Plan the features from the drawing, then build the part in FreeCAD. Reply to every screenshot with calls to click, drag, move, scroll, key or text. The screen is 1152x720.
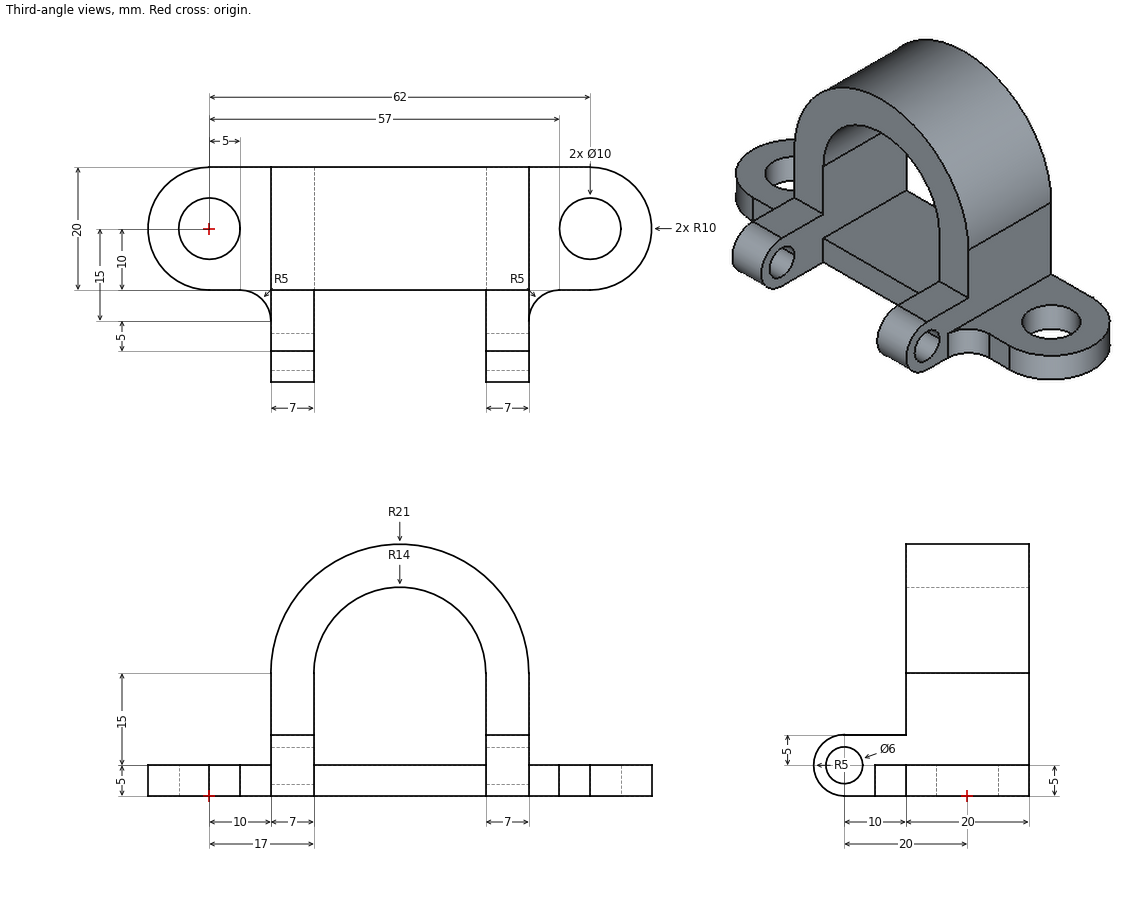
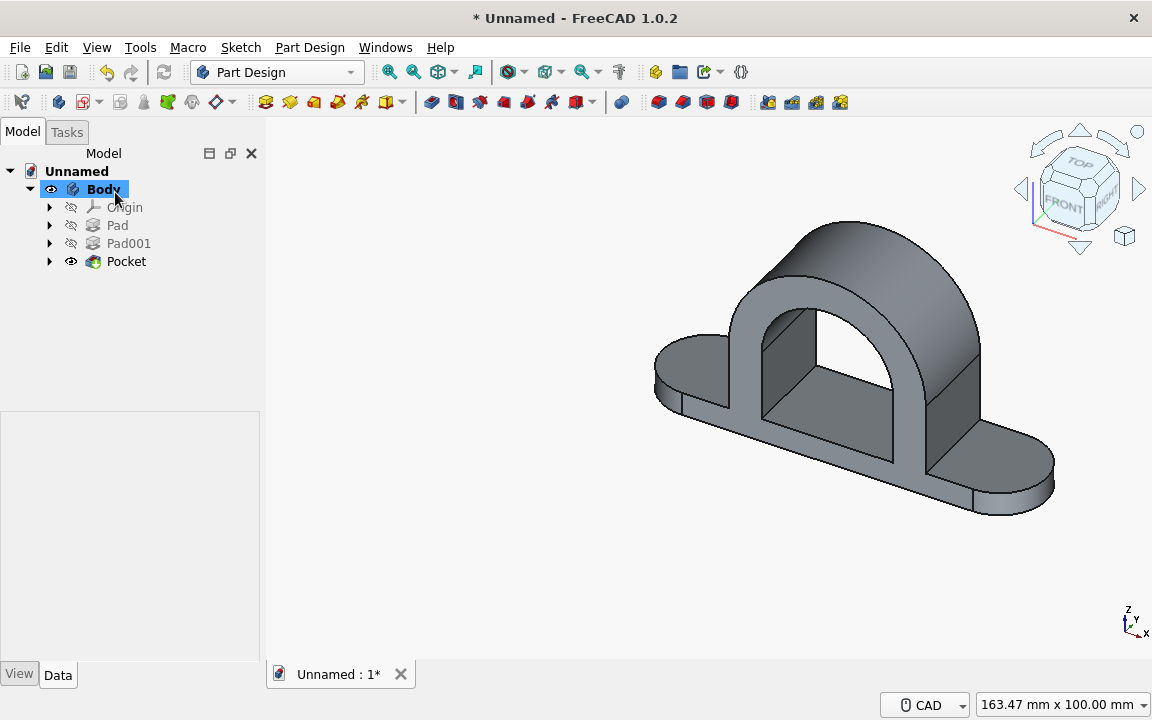
click(709, 365)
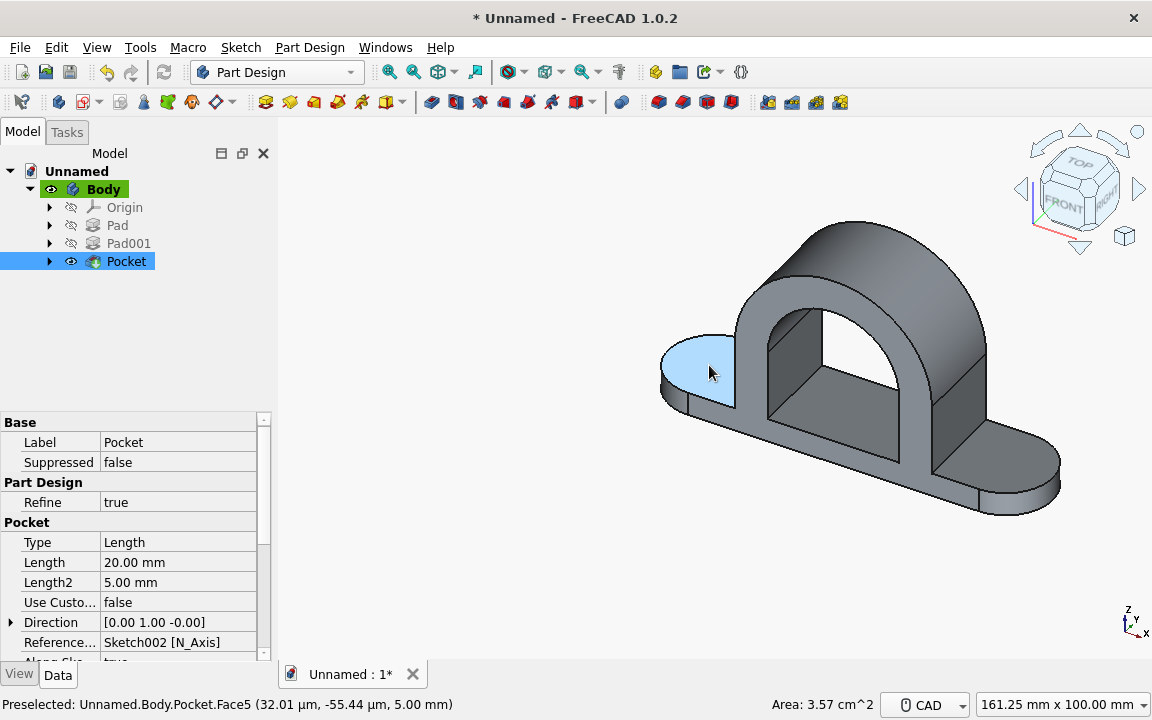
click(84, 102)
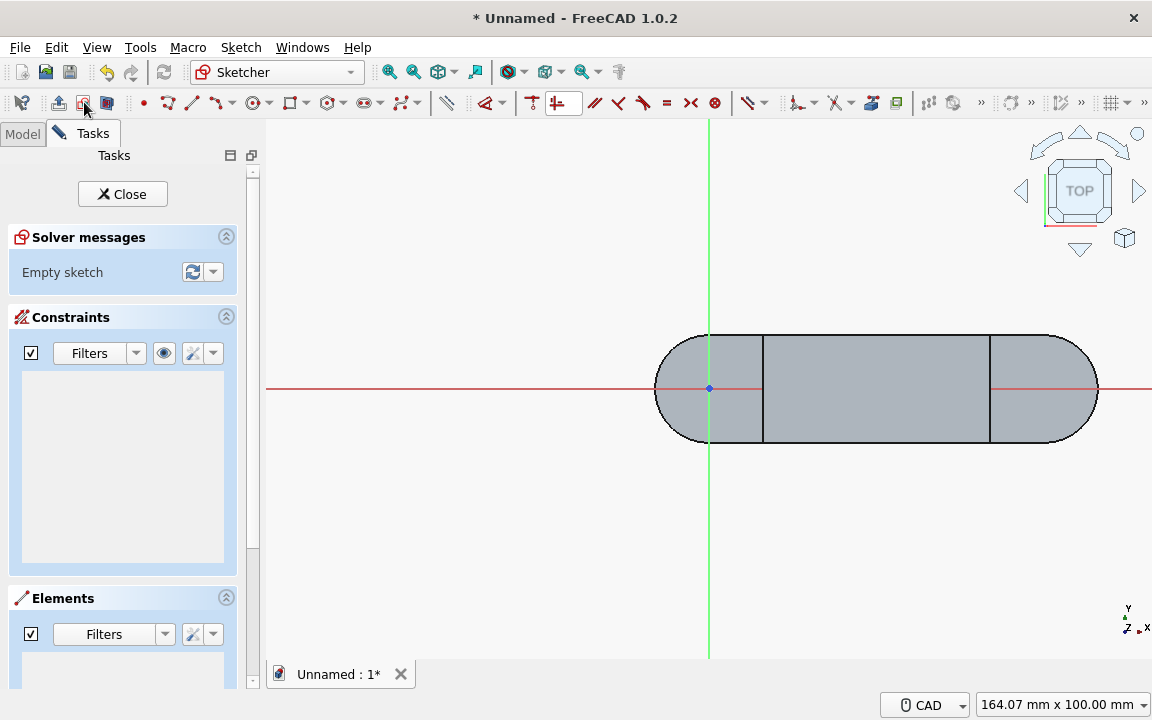
scroll(294, 389, down, 1)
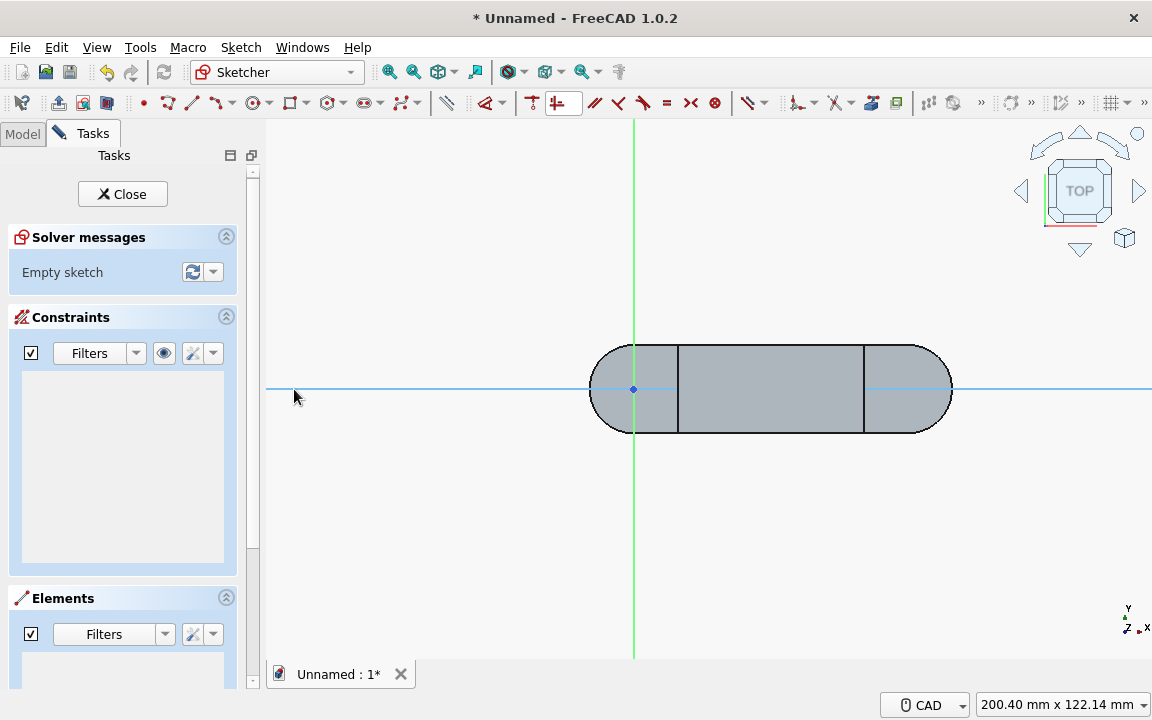
scroll(987, 389, up, 2)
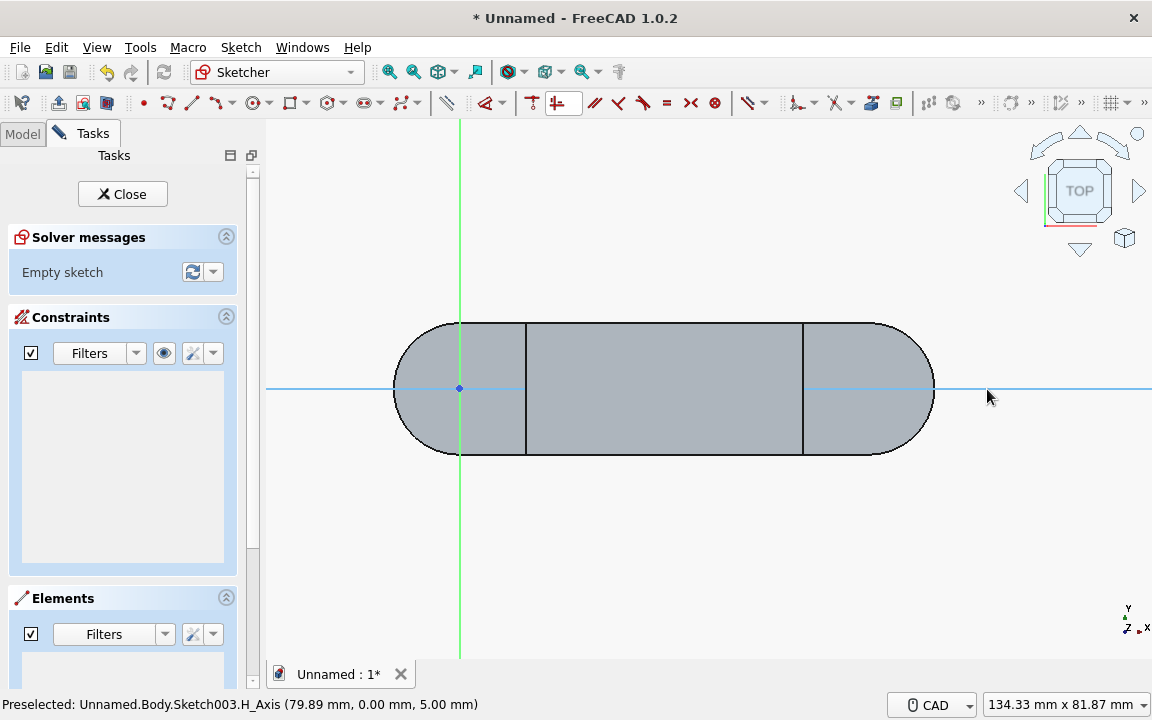
key(g)
key(c)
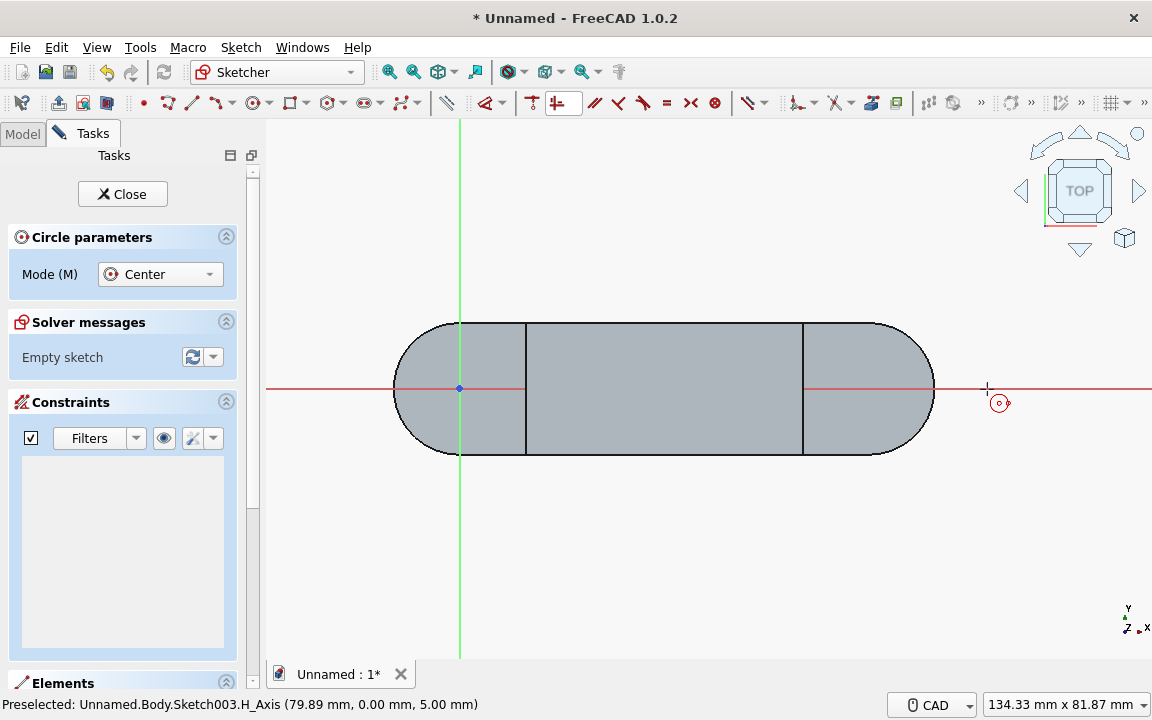
click(869, 389)
move(892, 366)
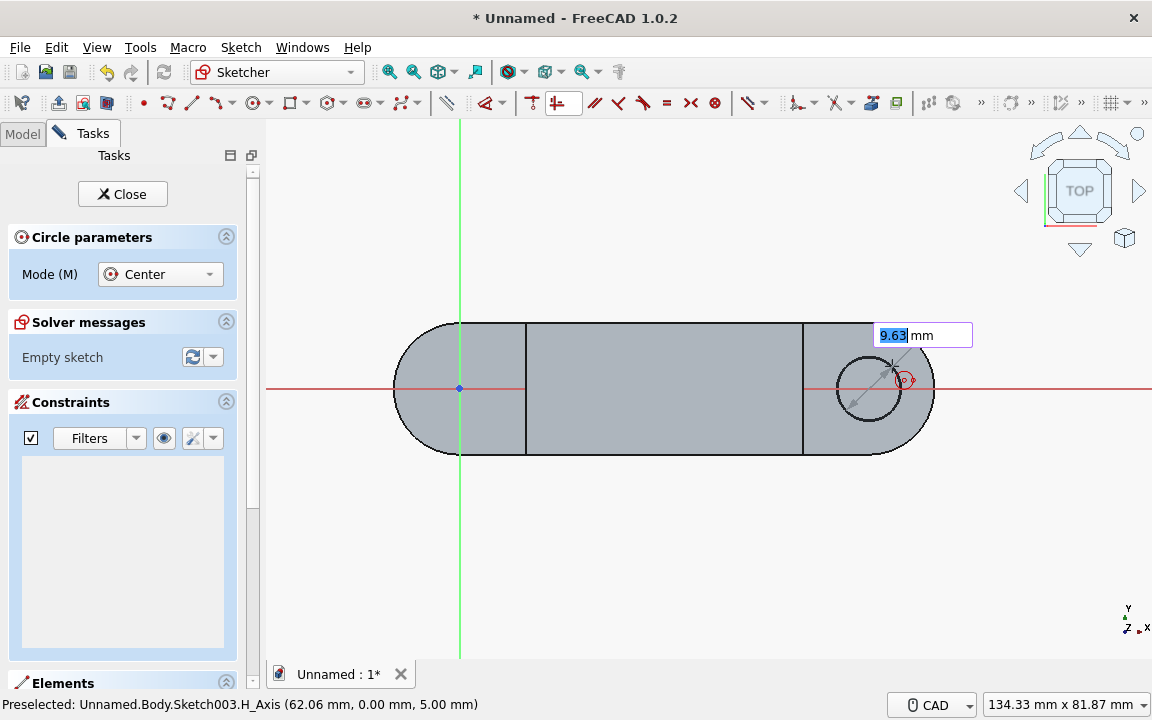
text(10)
key(Return)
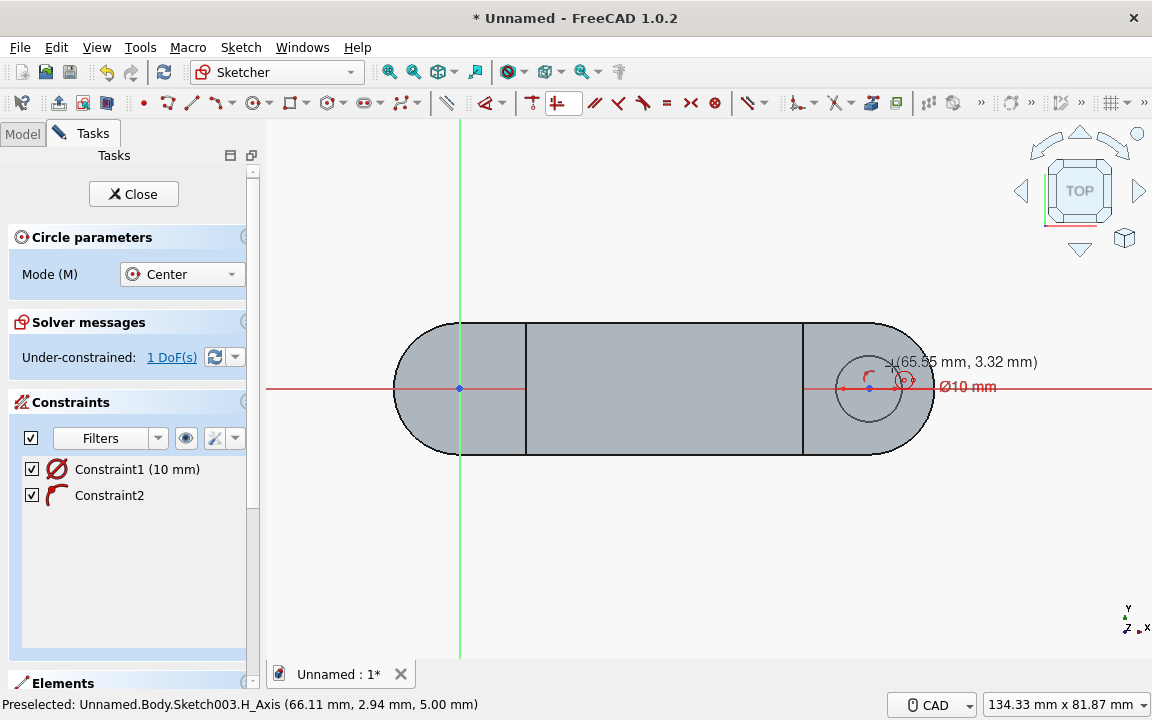
click(460, 389)
move(483, 366)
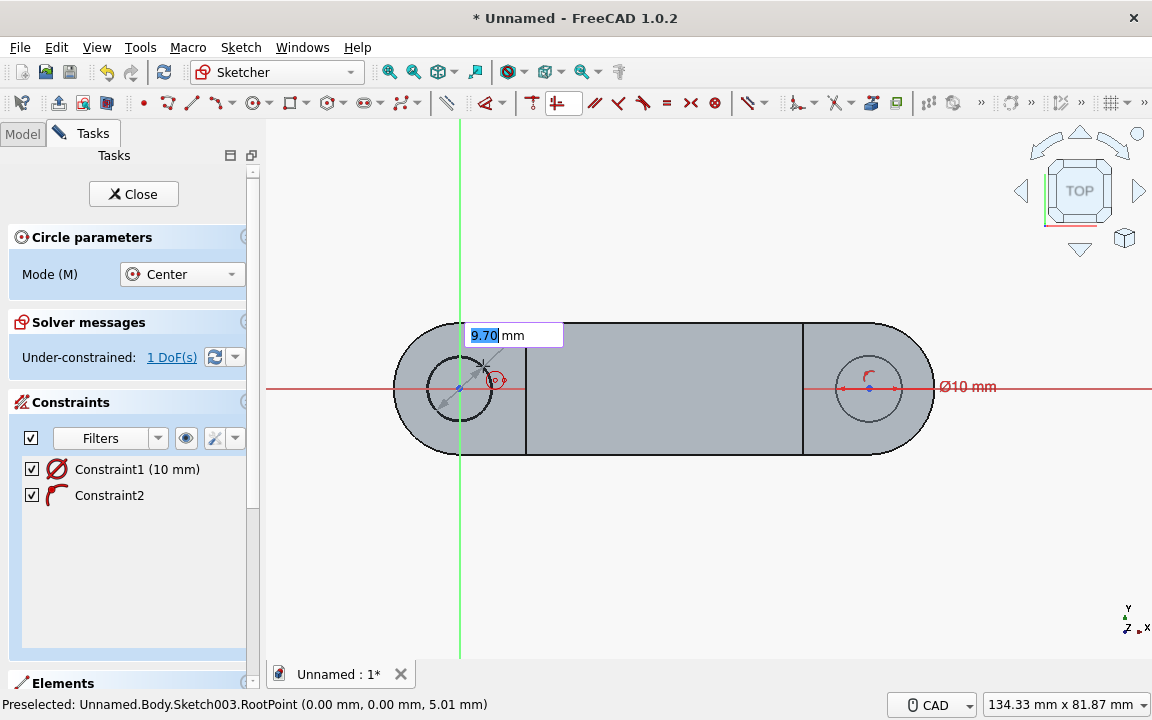
text(10)
key(Return)
key(Escape)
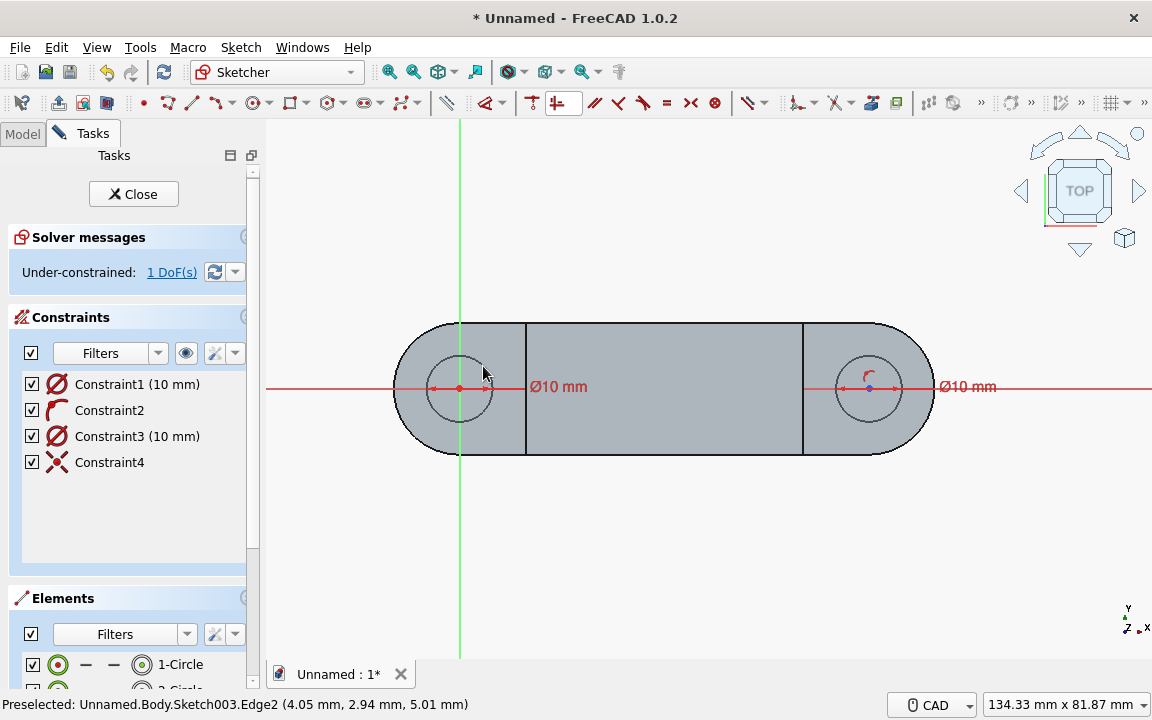
click(486, 104)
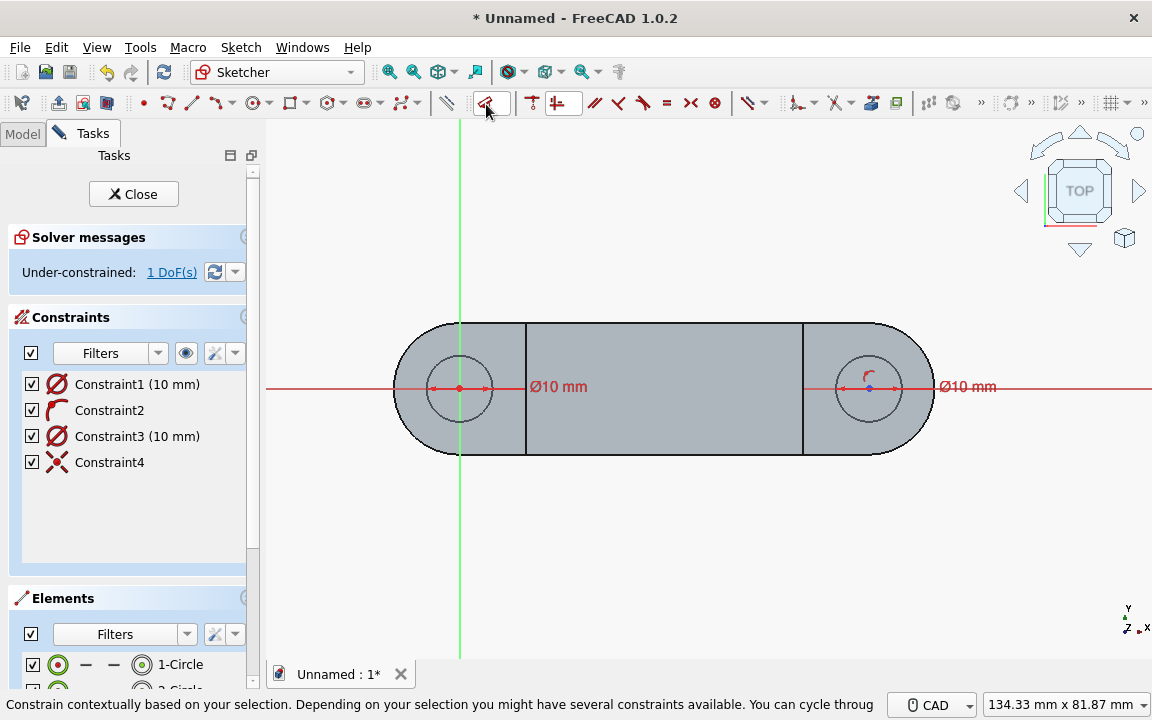
click(869, 389)
click(664, 423)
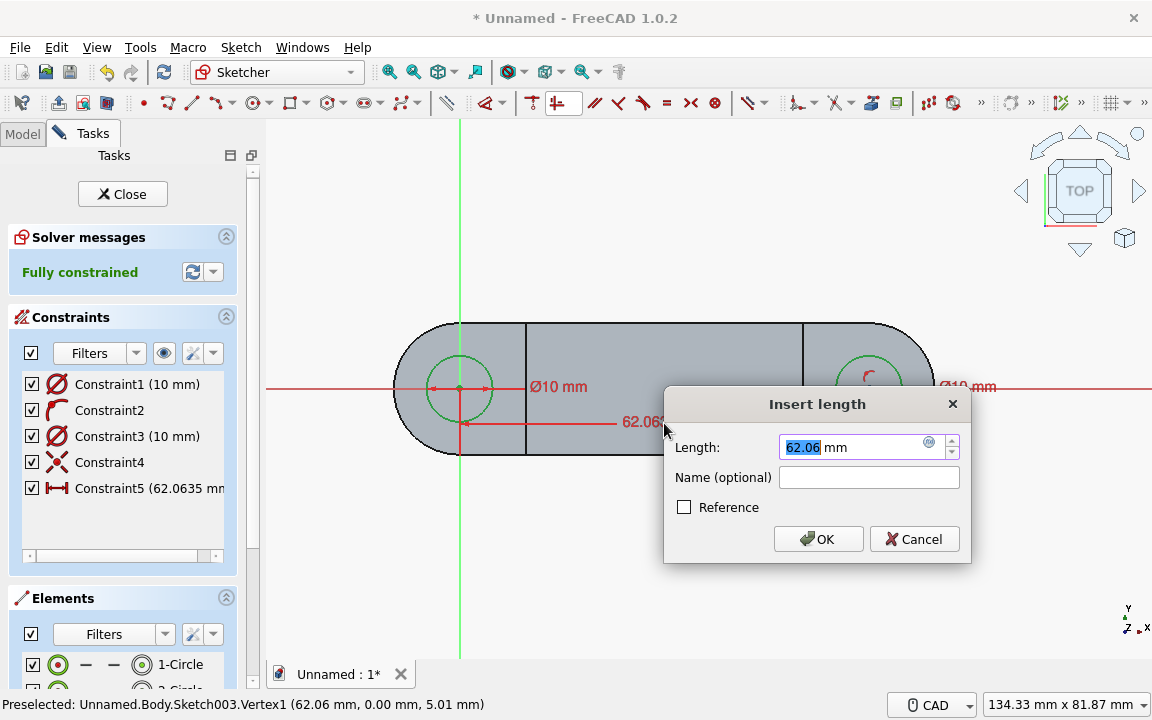
text(62)
key(Return)
key(Escape)